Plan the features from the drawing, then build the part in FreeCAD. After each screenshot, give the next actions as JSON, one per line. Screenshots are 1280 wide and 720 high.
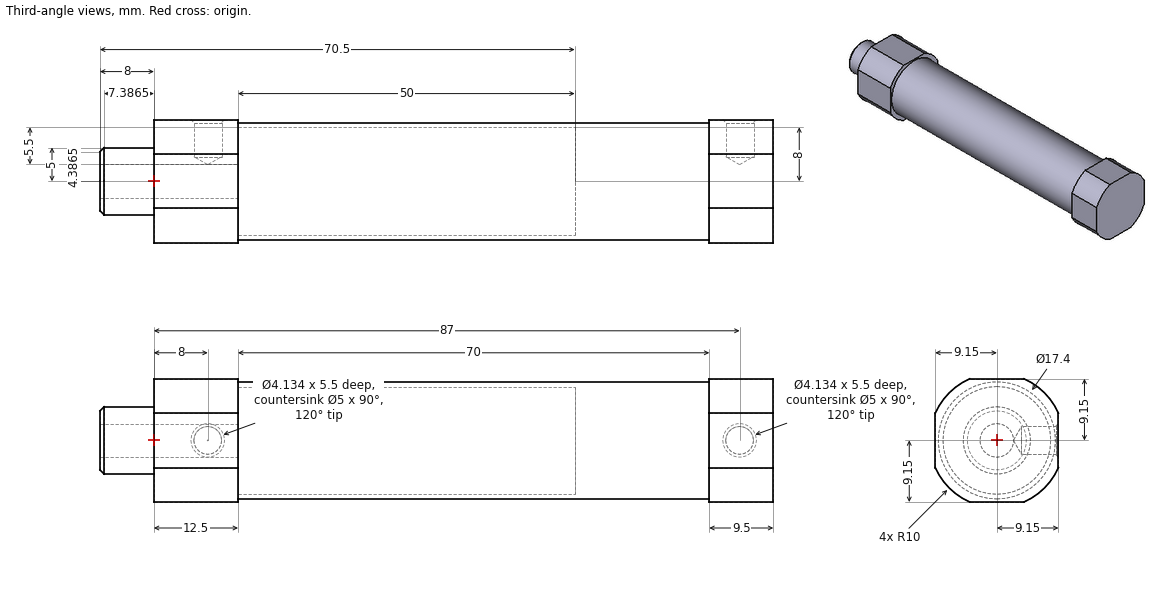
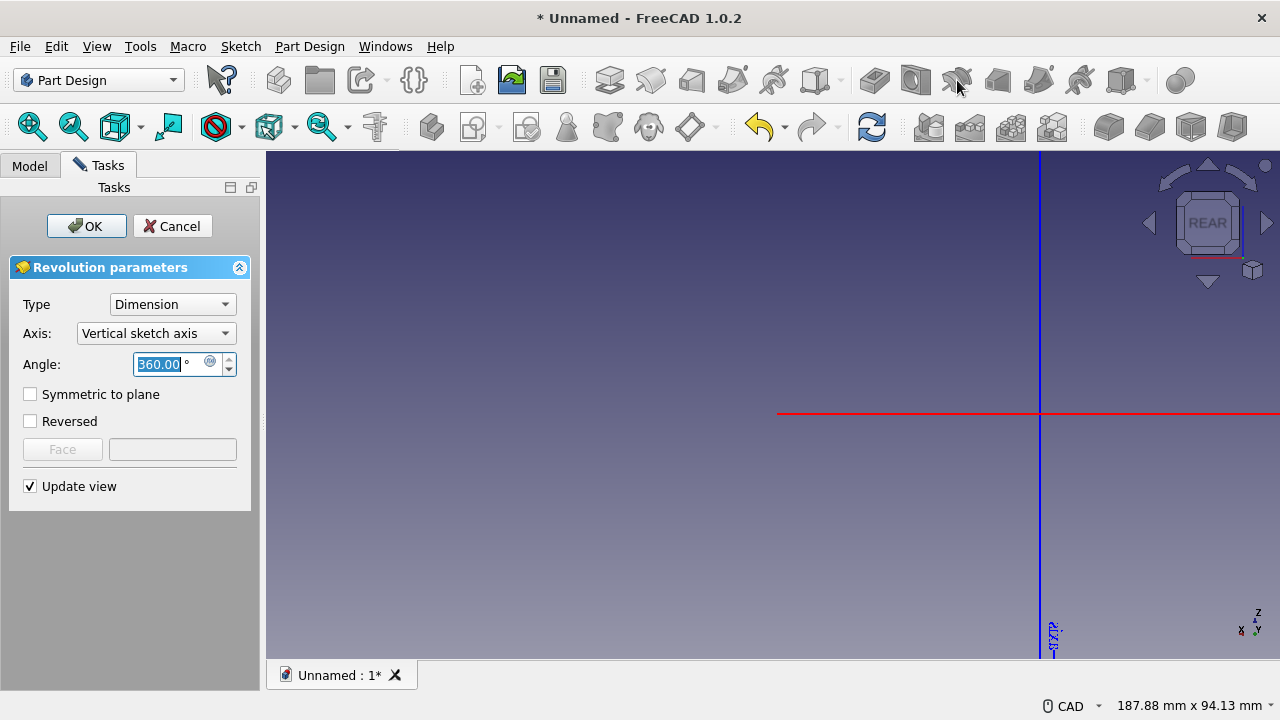
{"action": "left_click", "coordinate": [157, 334]}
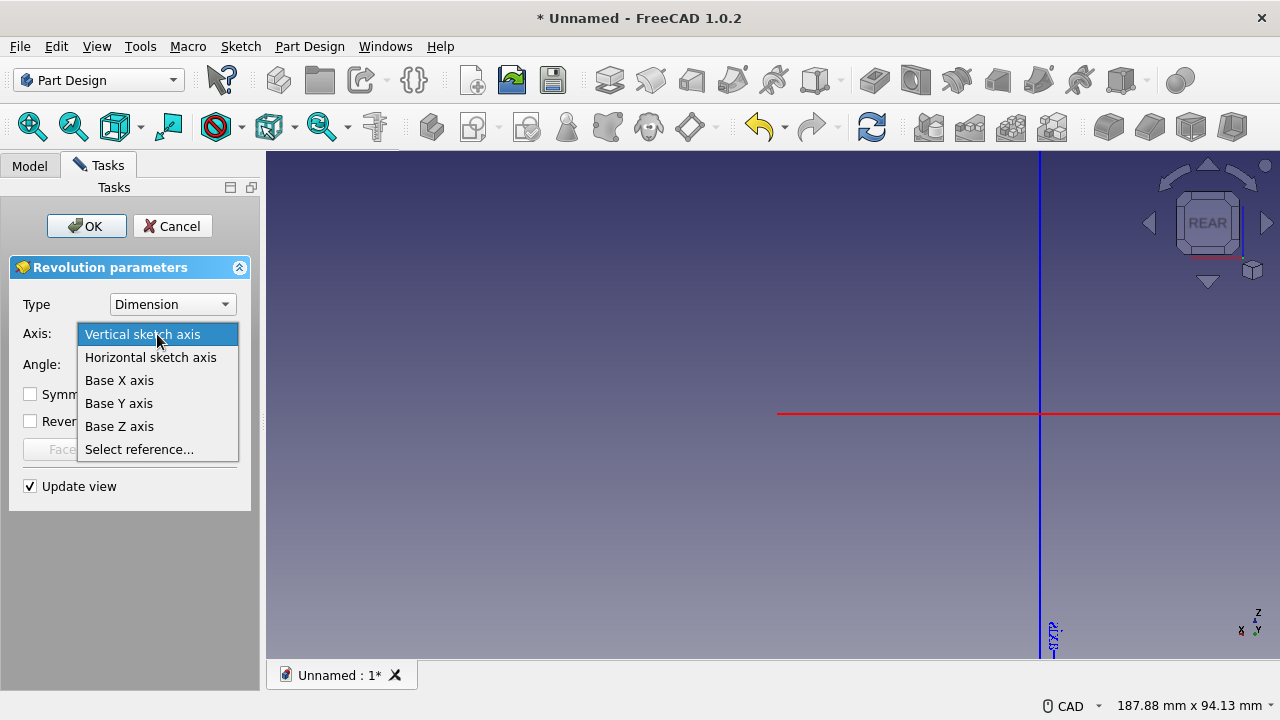
{"action": "left_click", "coordinate": [156, 358]}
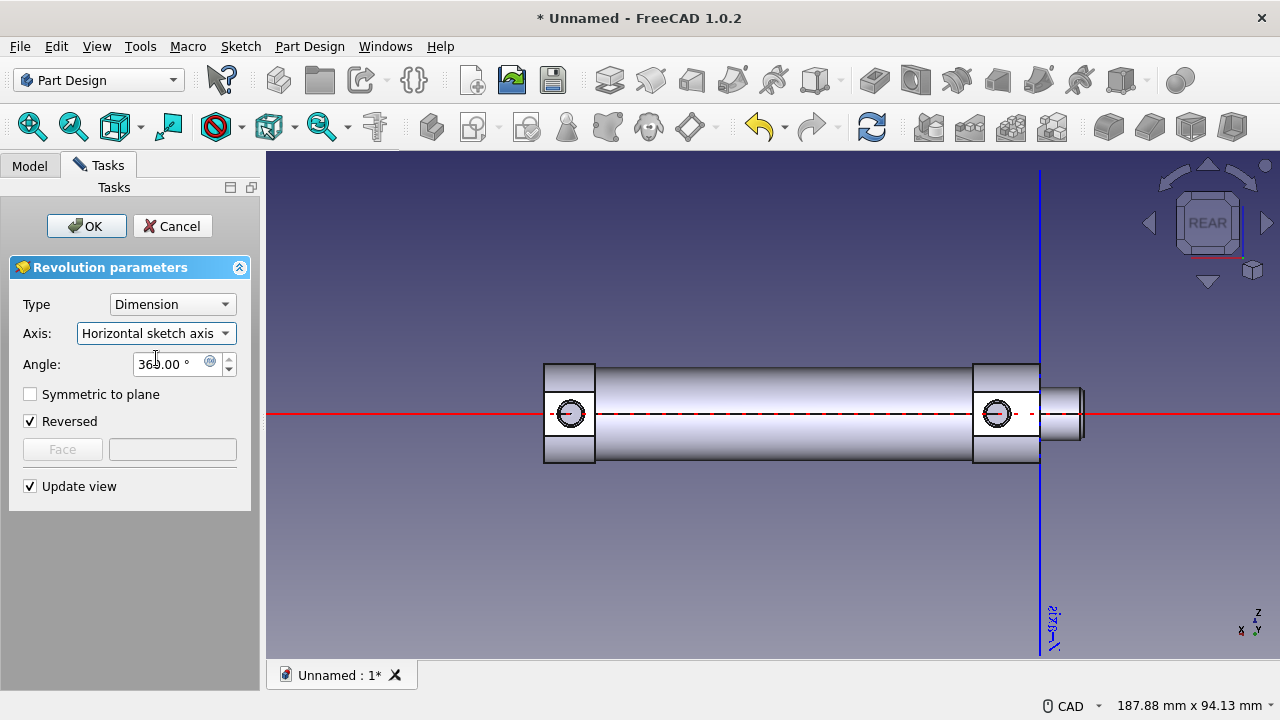
{"action": "left_click", "coordinate": [87, 226]}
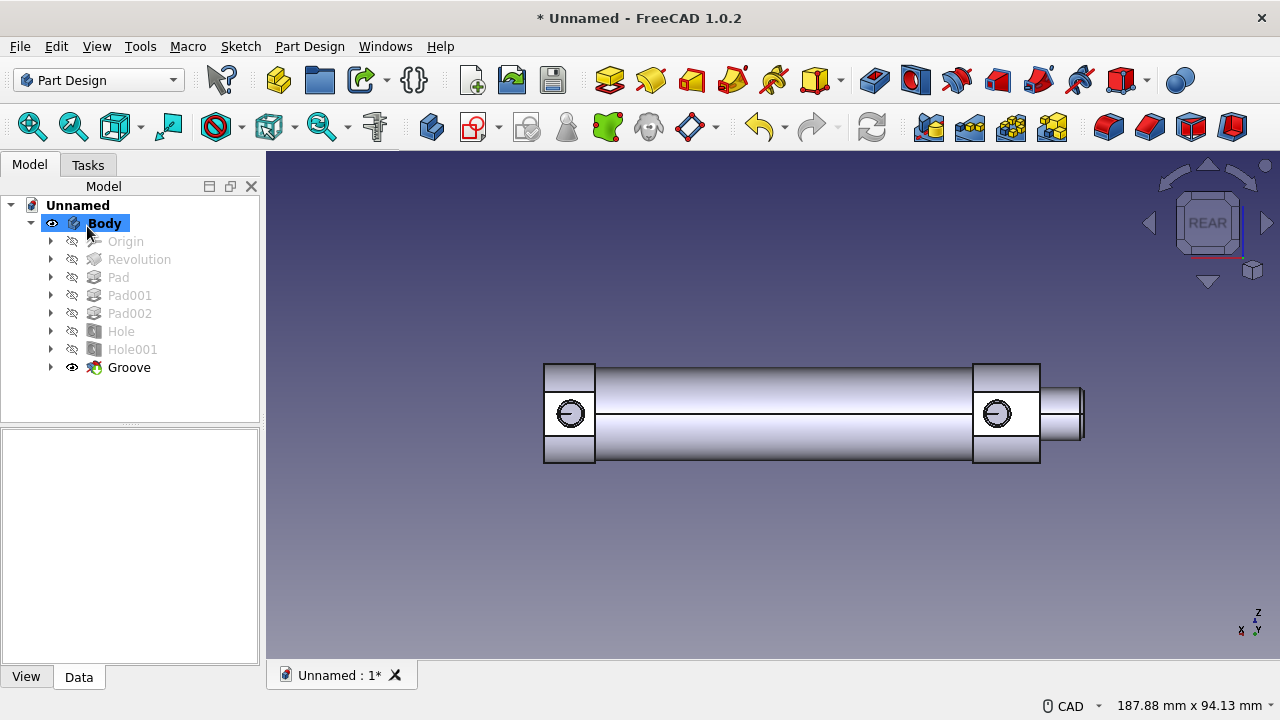
{"action": "key", "text": "0"}